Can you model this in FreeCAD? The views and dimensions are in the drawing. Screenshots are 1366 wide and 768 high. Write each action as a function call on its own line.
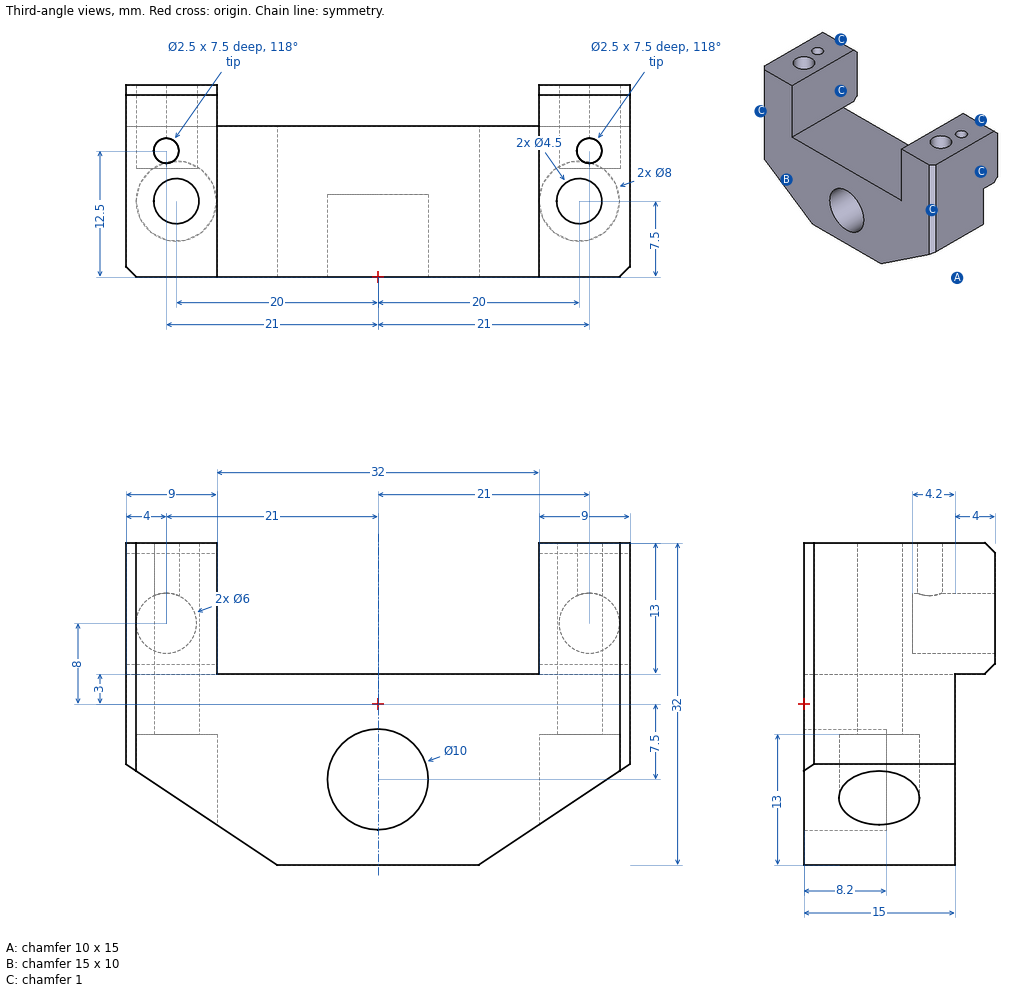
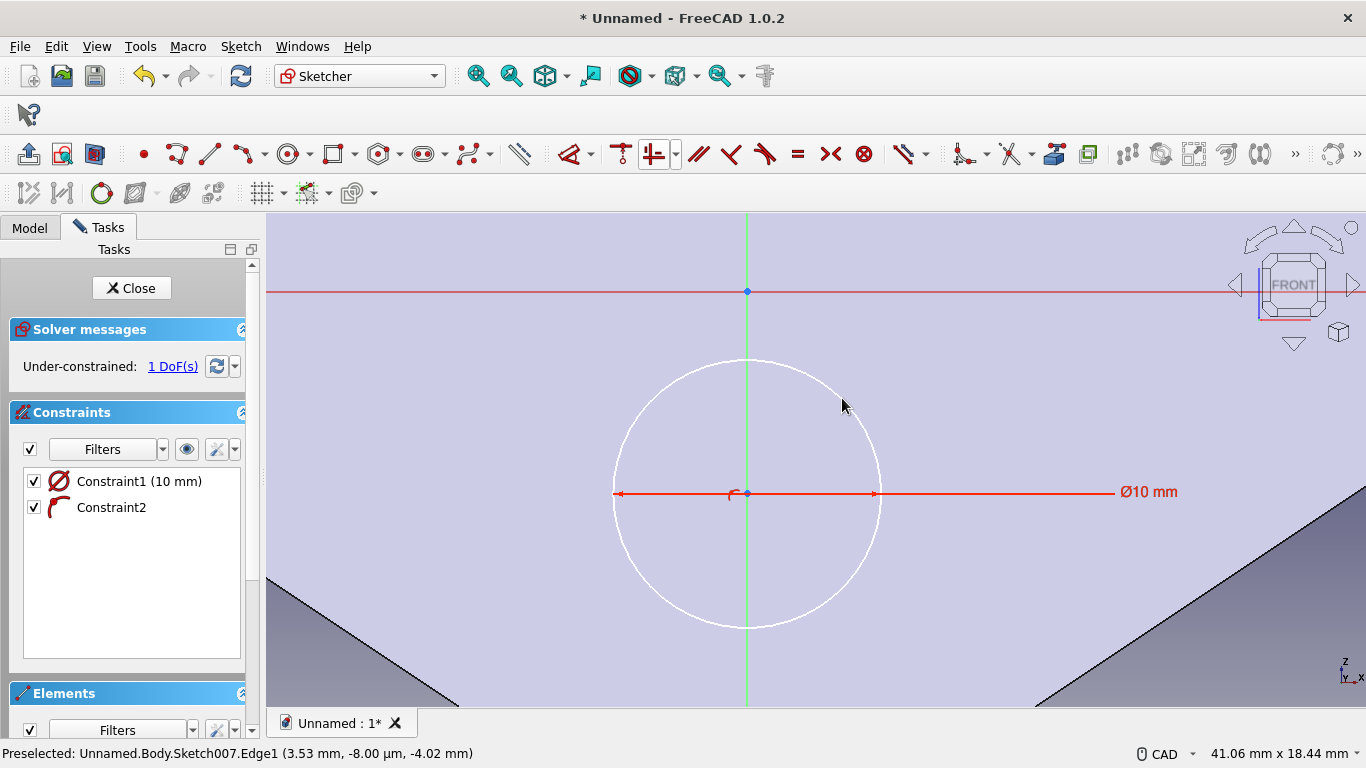
click(568, 154)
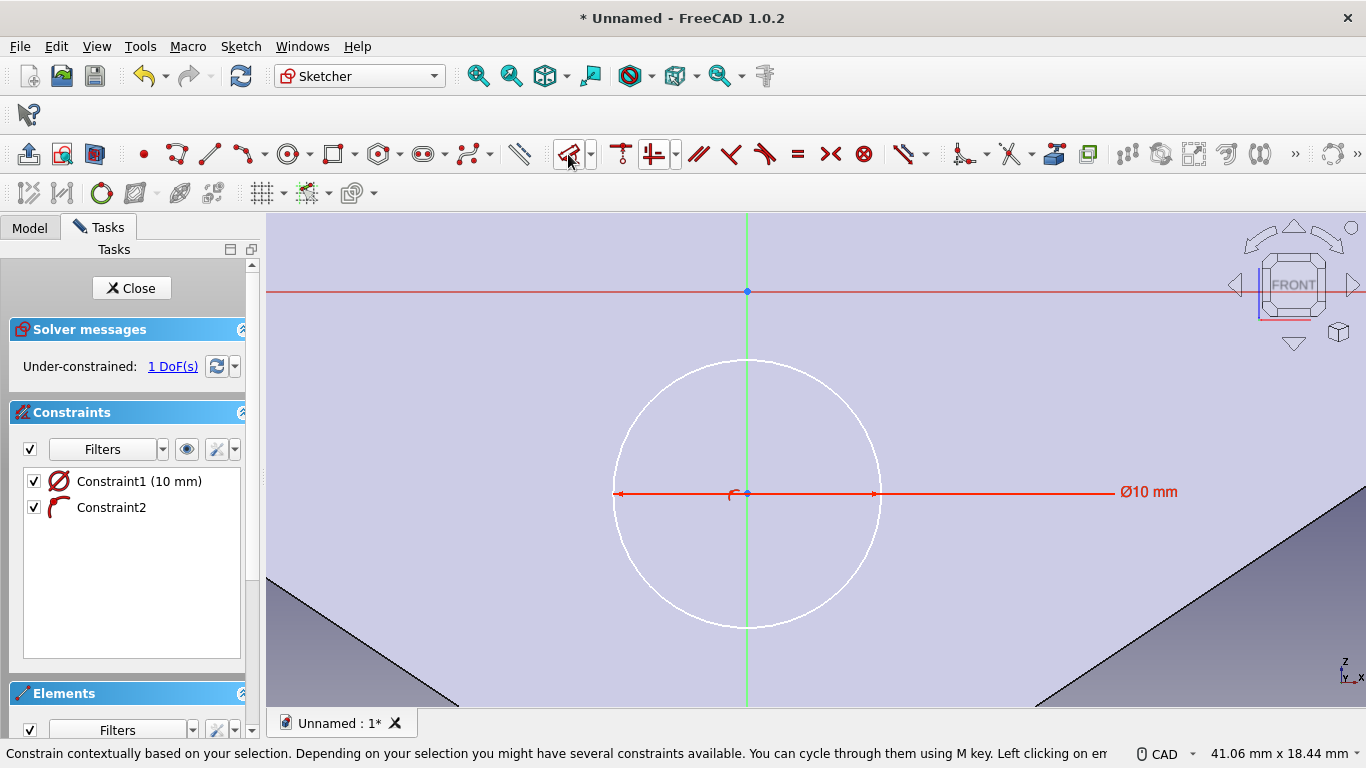
click(747, 494)
click(781, 393)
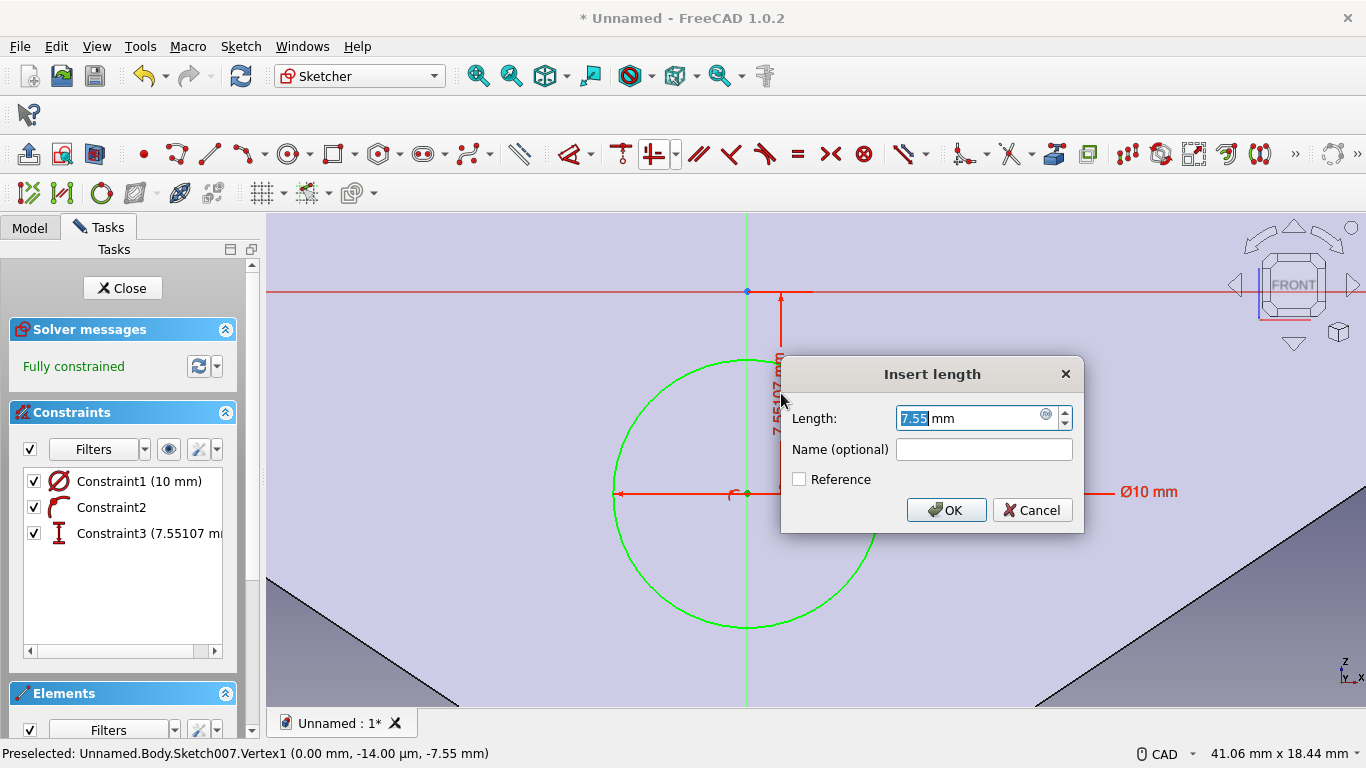
text(7.5)
key(Return)
key(Escape)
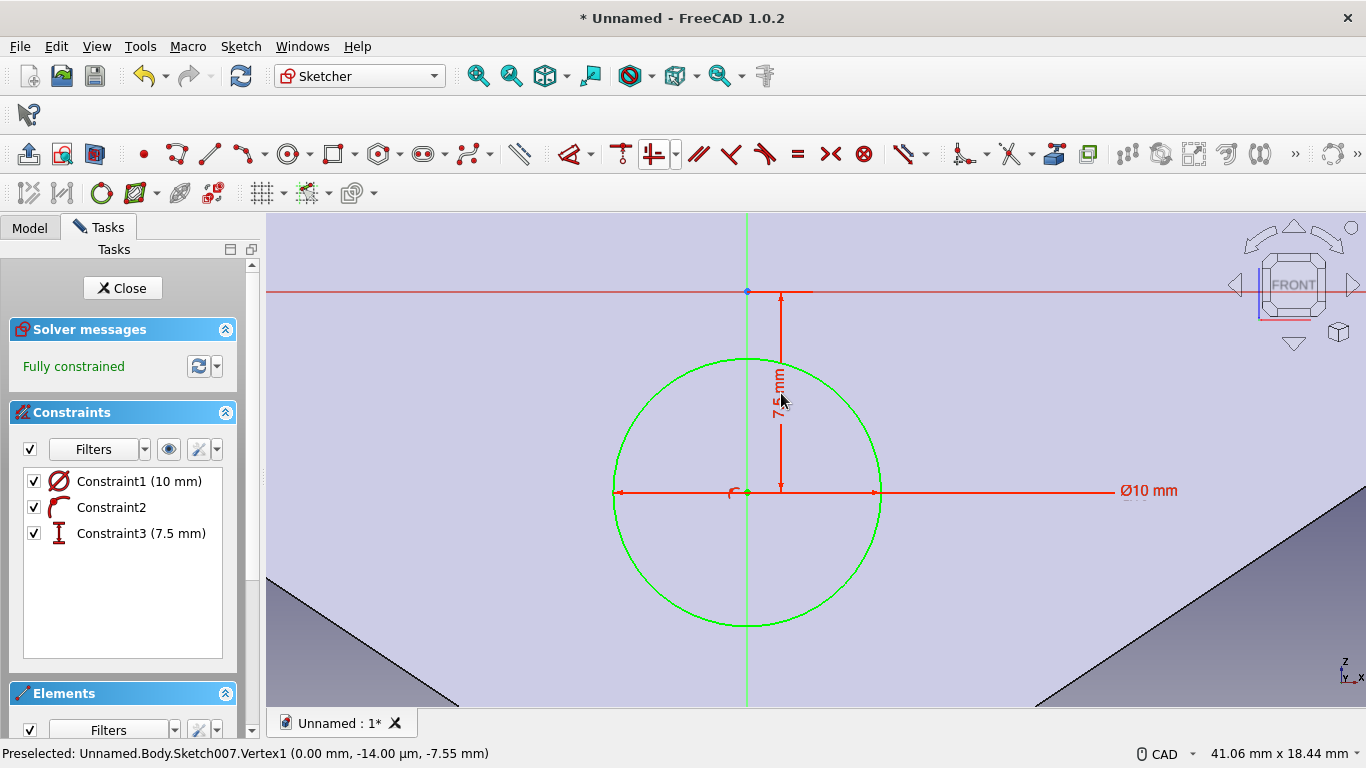
click(123, 288)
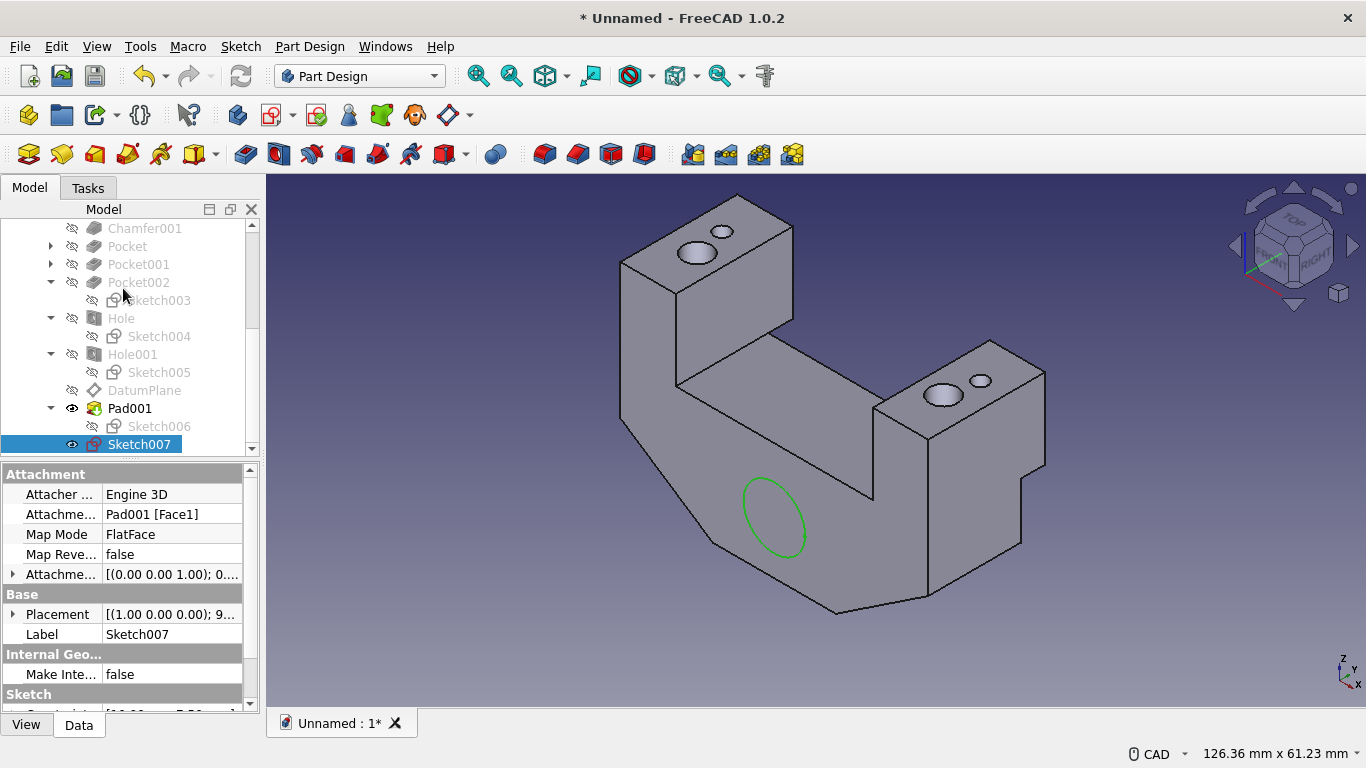
click(246, 154)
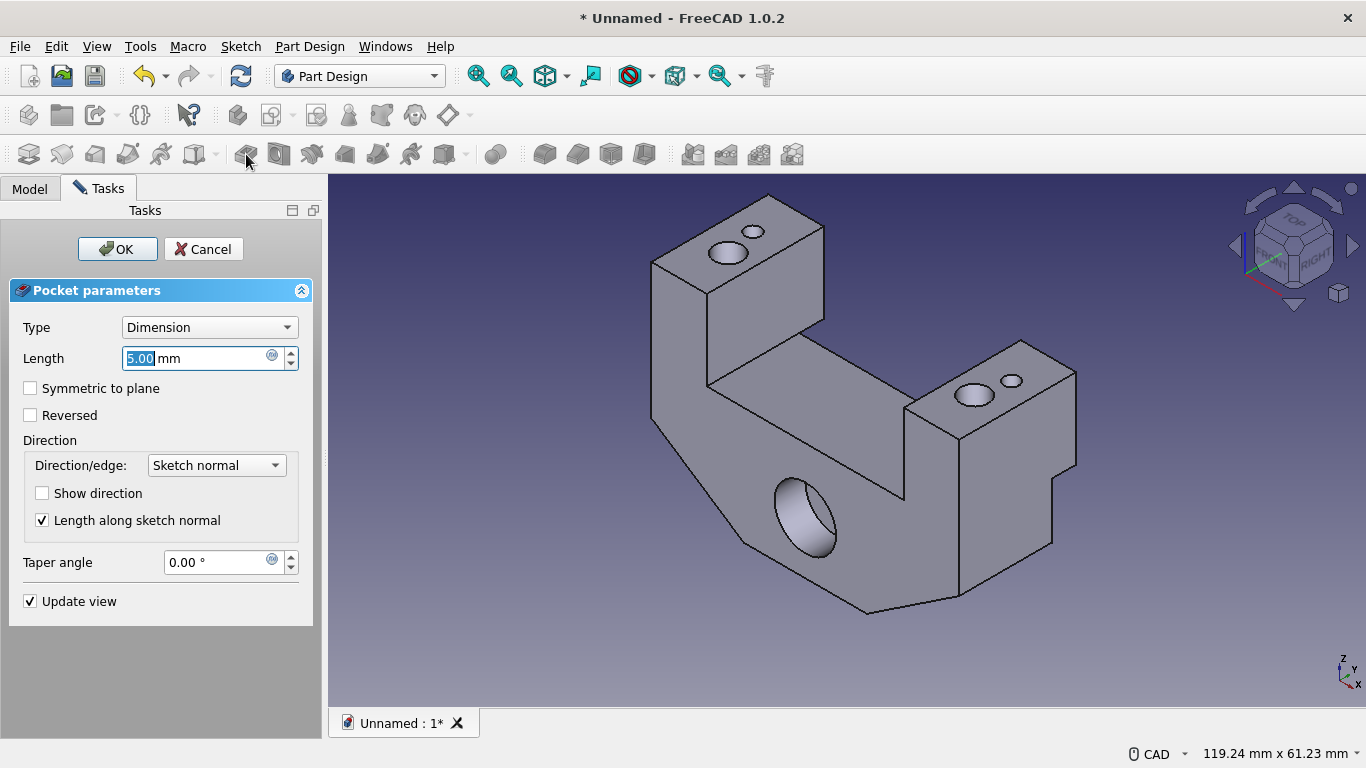
text(8.2)
key(Tab)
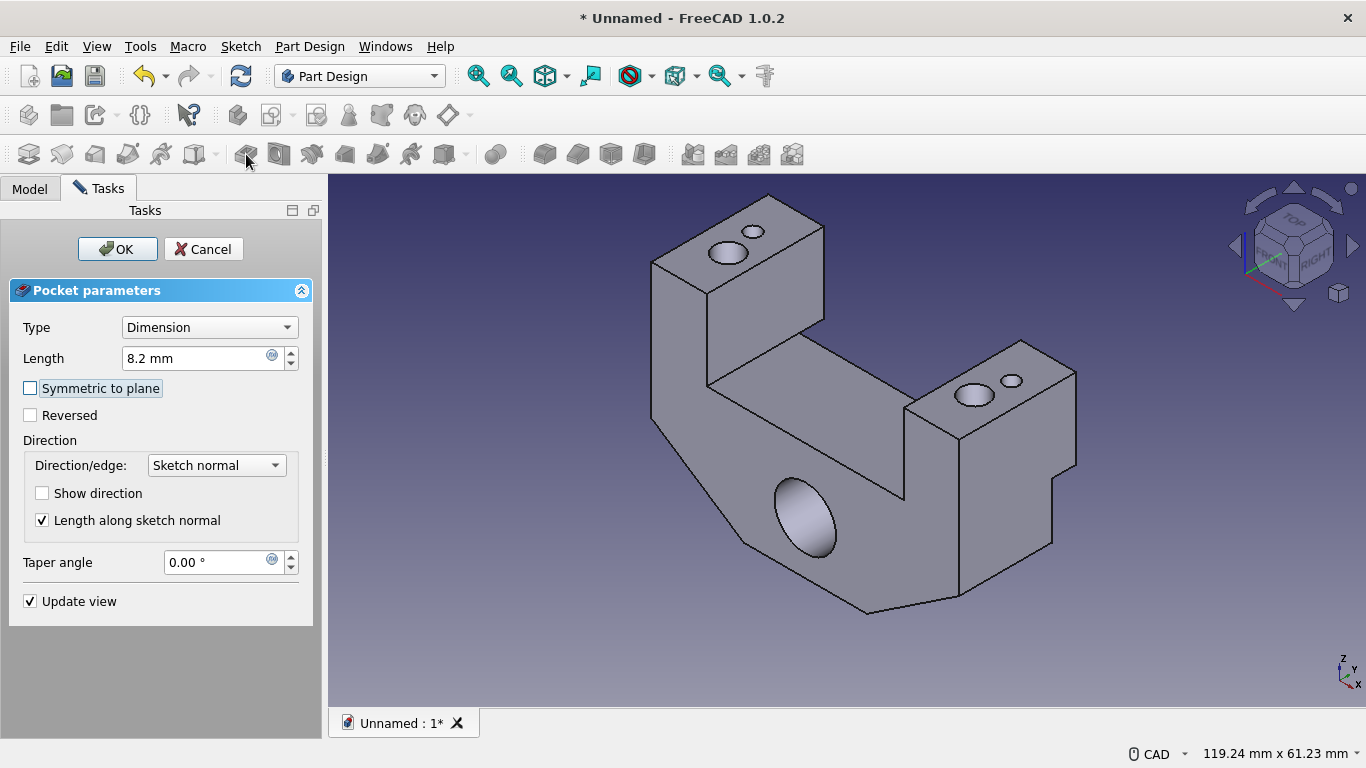
click(118, 249)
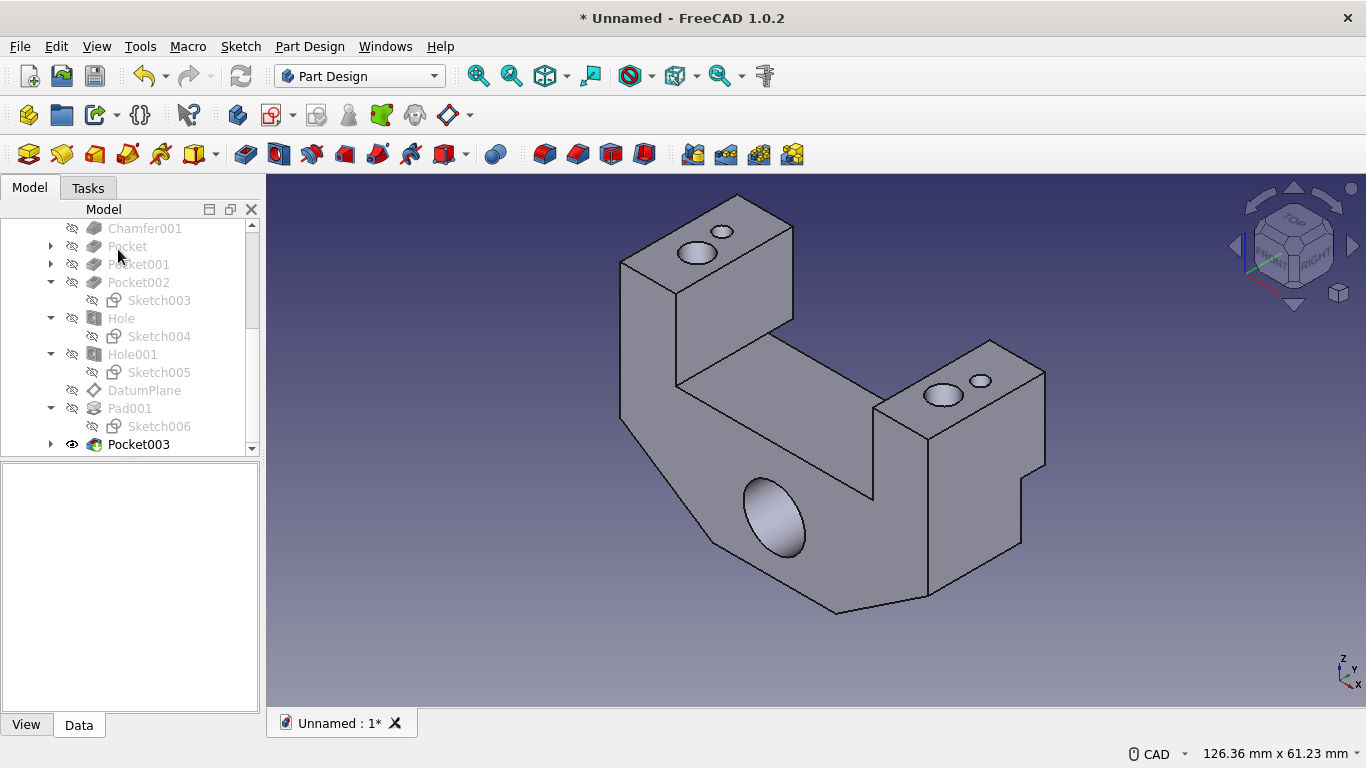
click(928, 517)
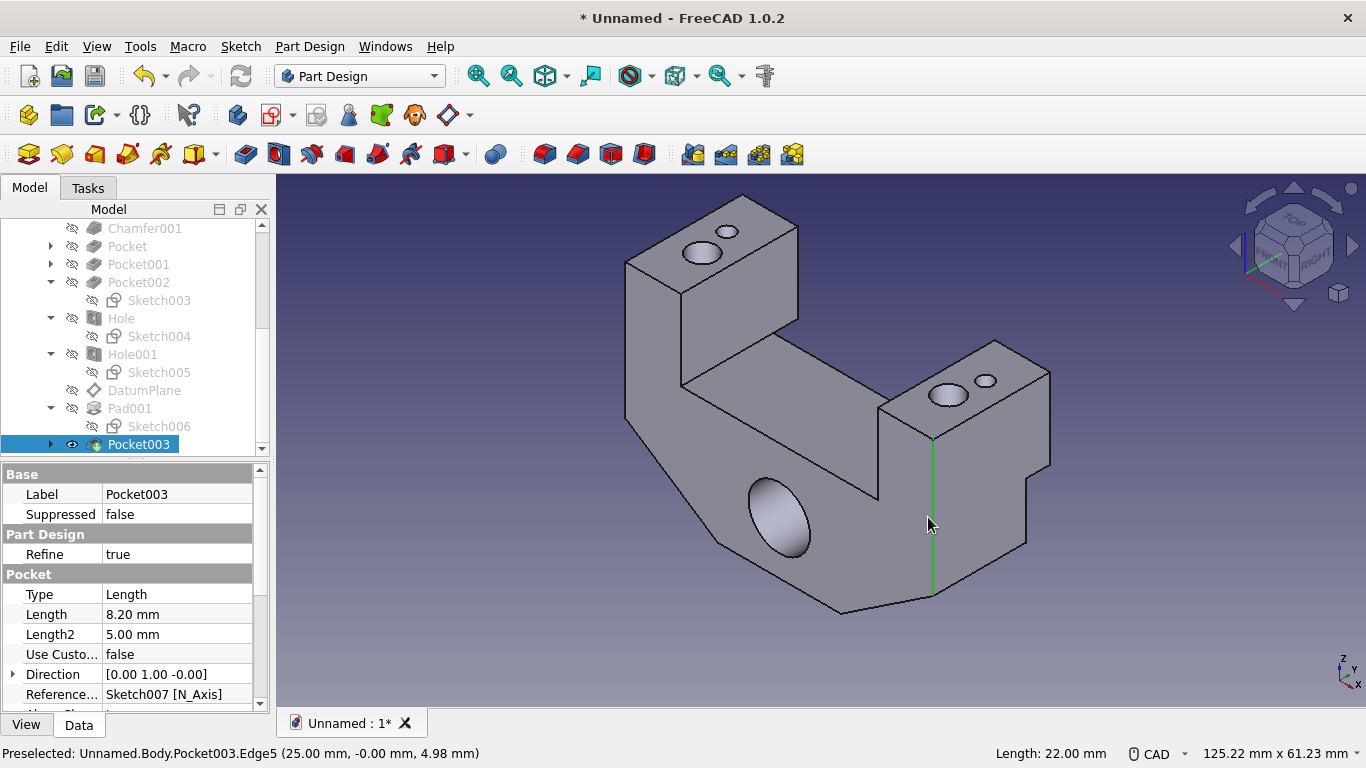
key(2)